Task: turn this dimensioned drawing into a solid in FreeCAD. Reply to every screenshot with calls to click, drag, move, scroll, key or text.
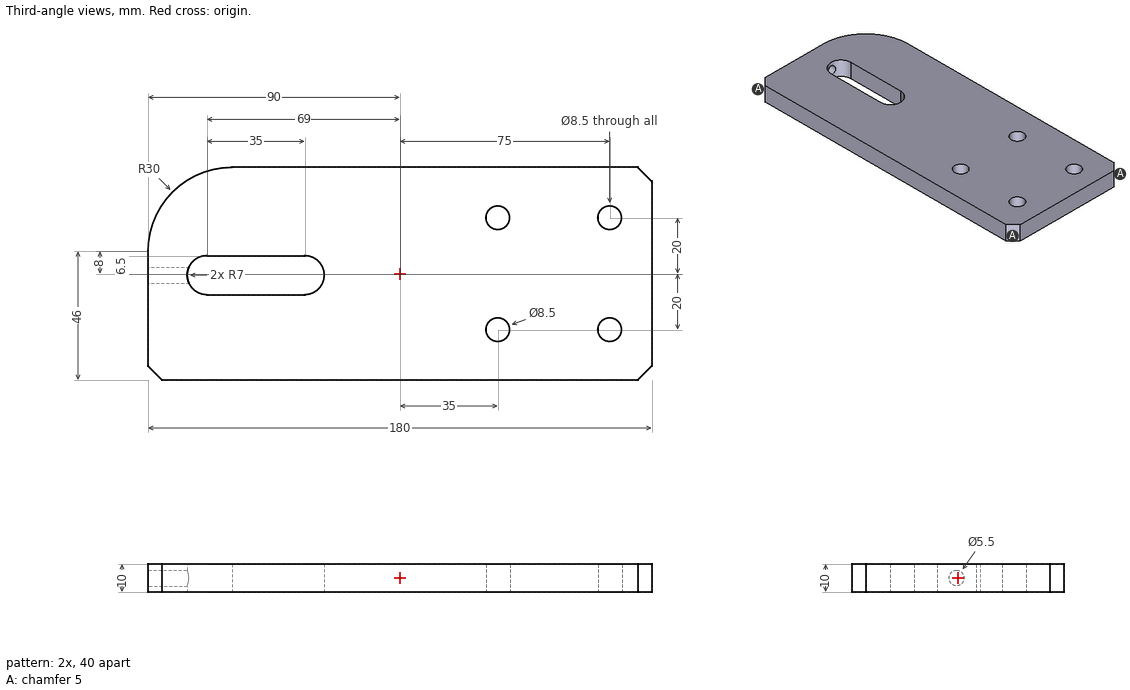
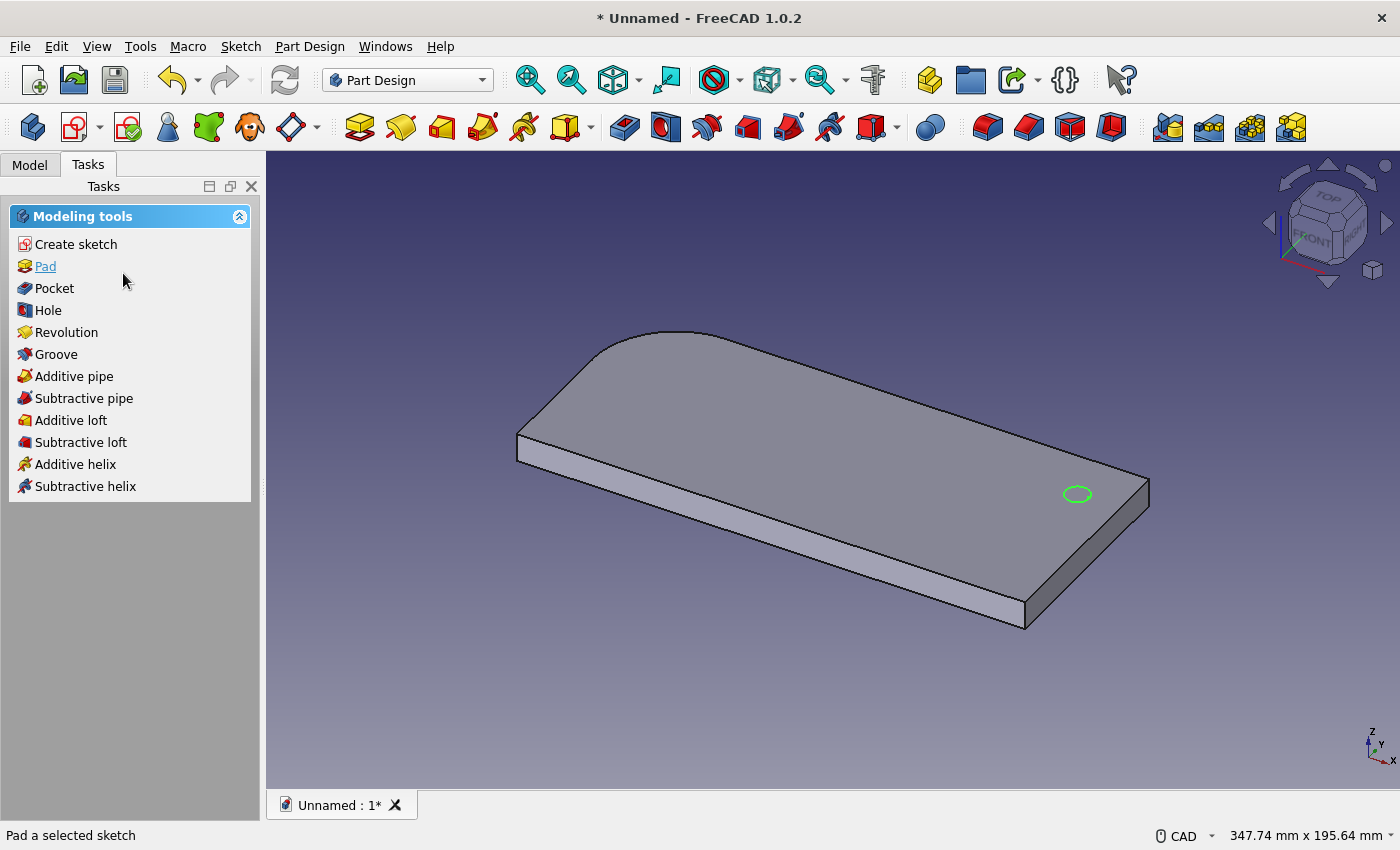
click(666, 128)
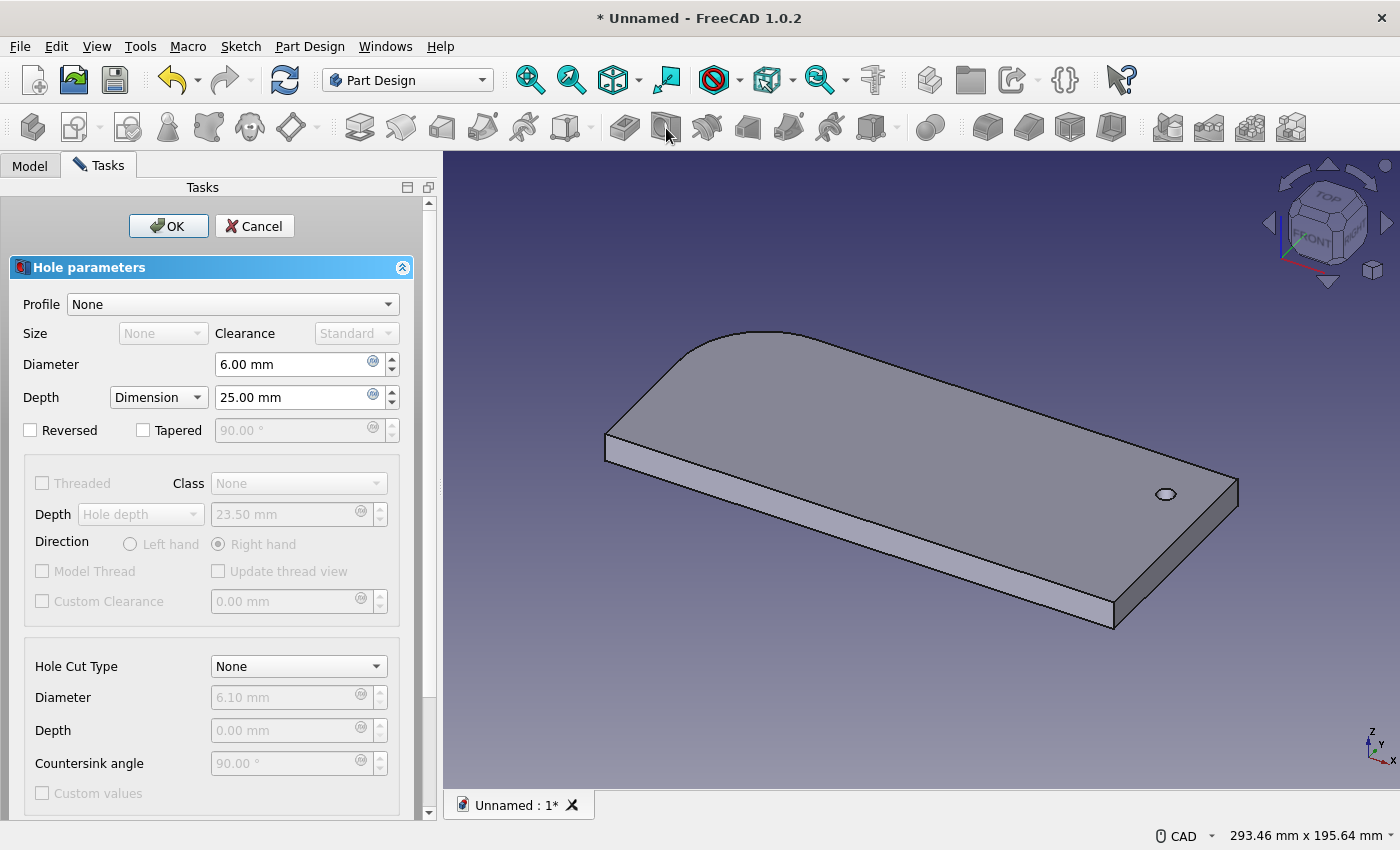
triple_click(300, 364)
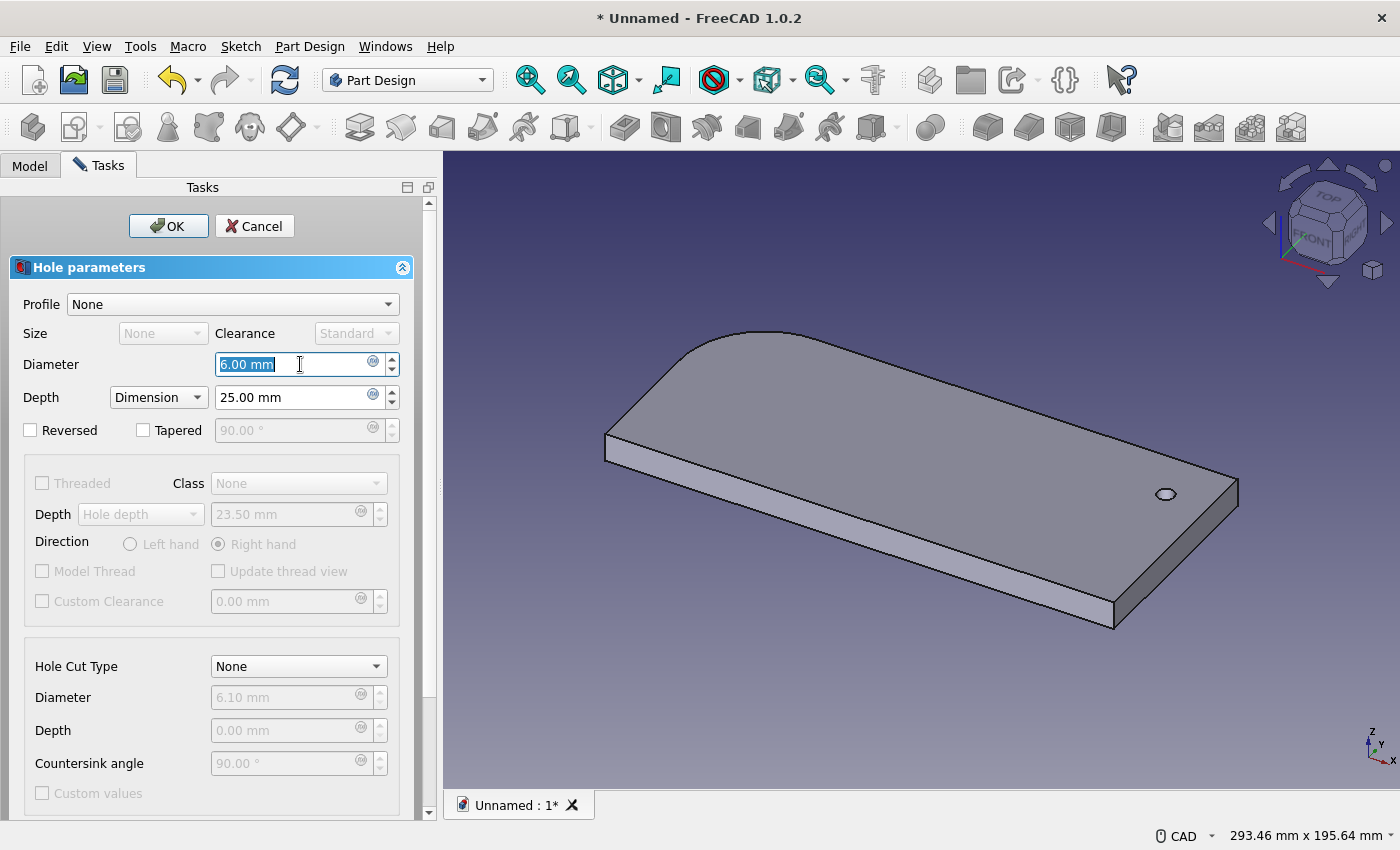
text(8.5)
key(Tab)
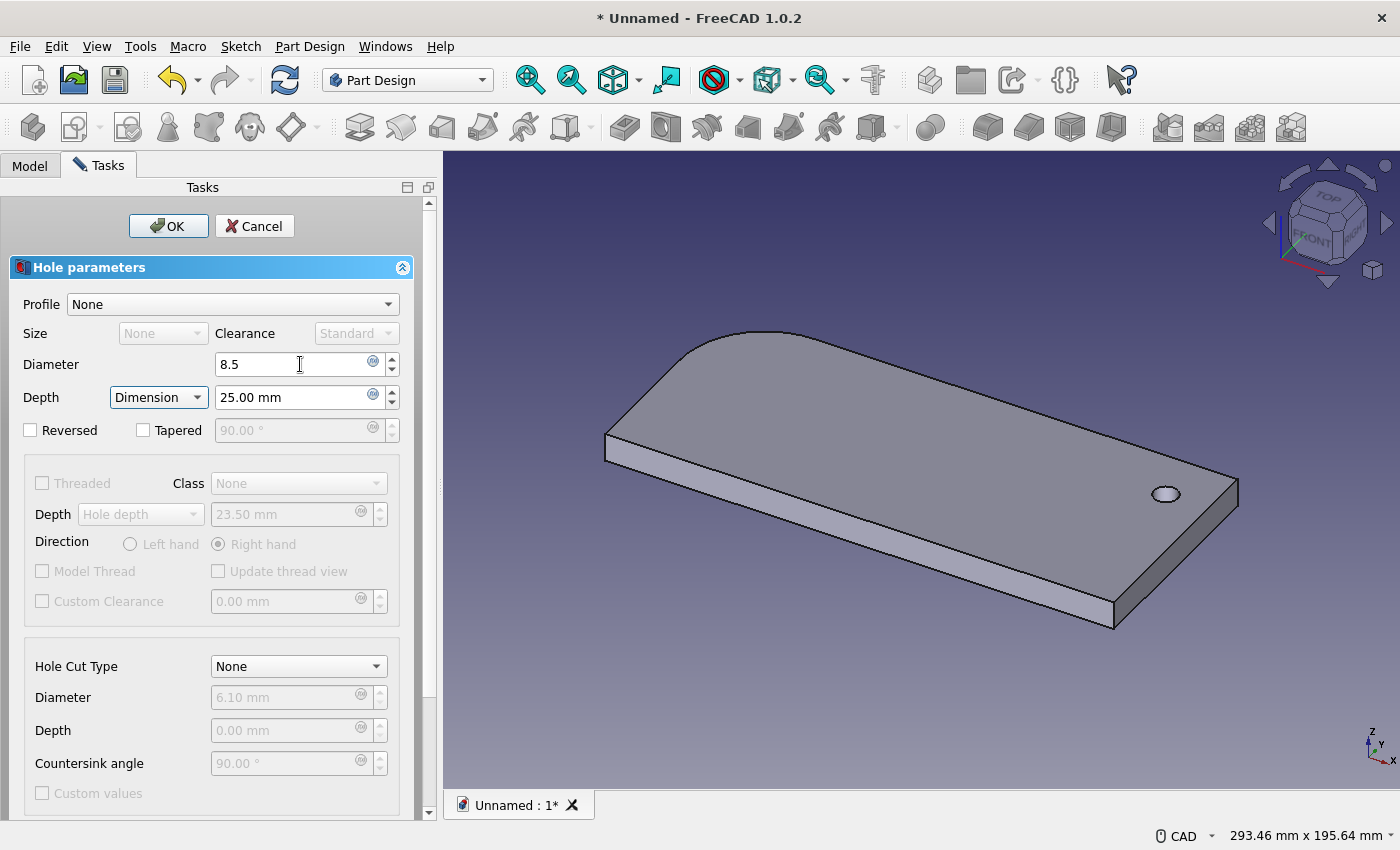
click(160, 398)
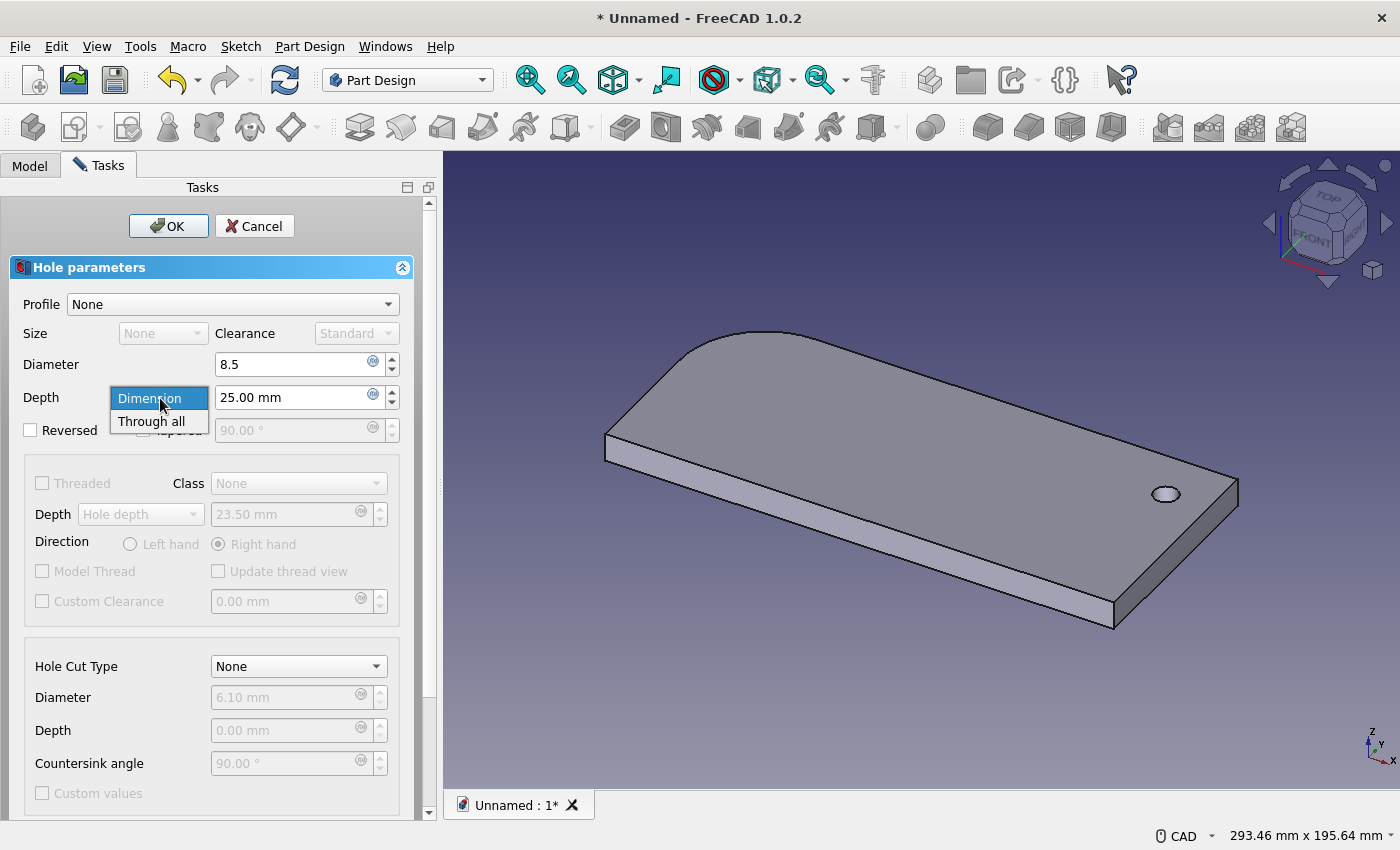
click(158, 422)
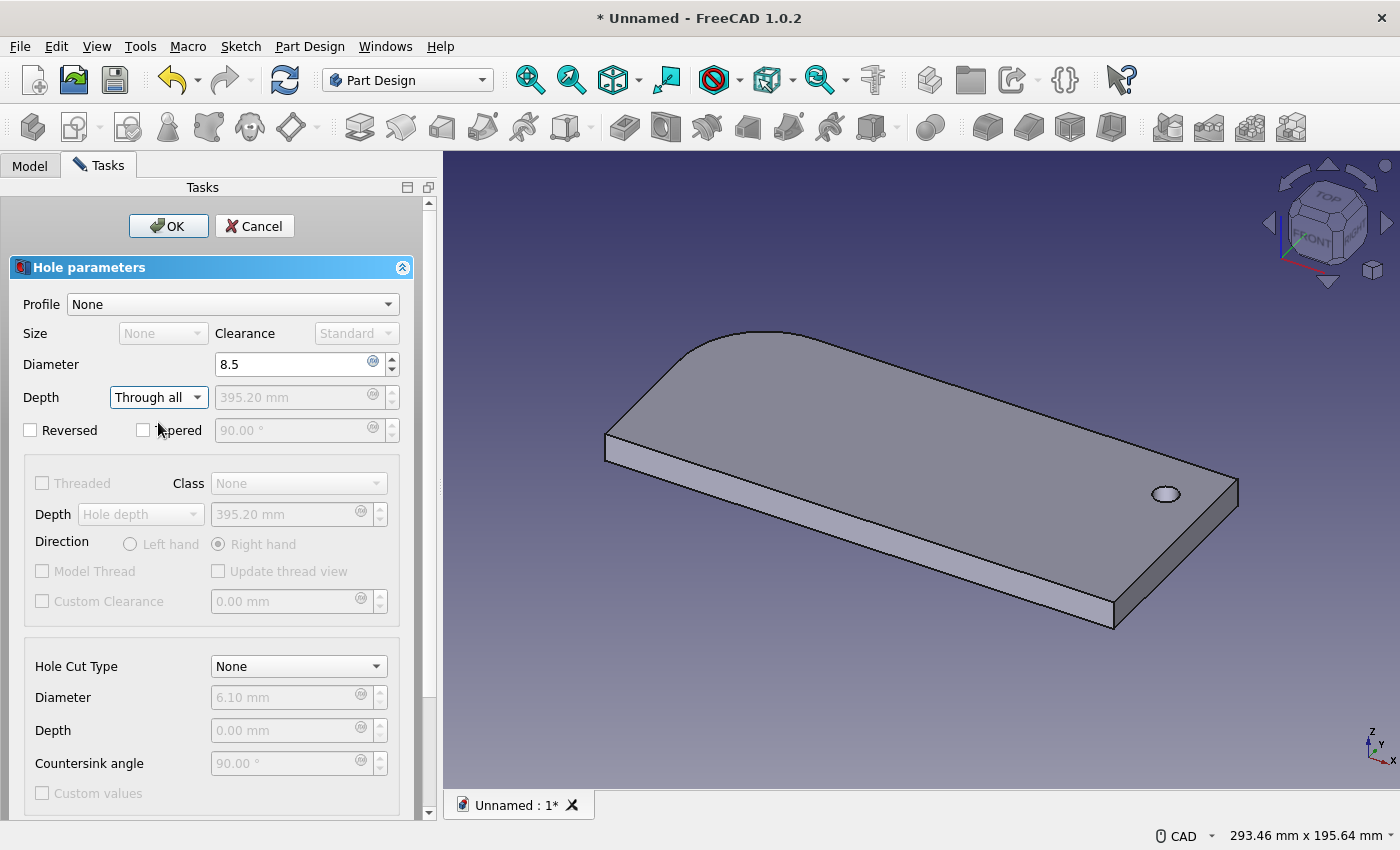
click(169, 226)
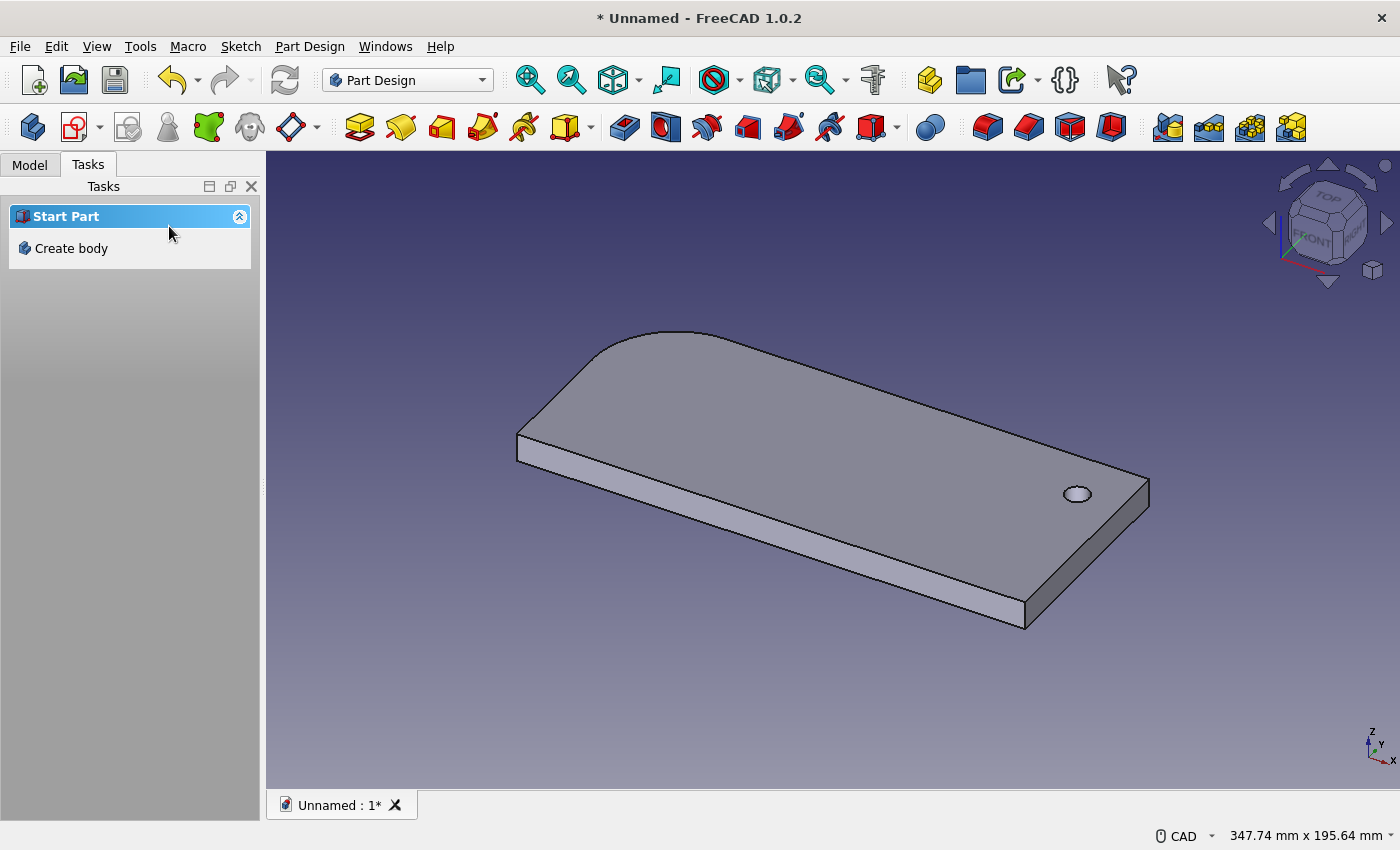
click(30, 164)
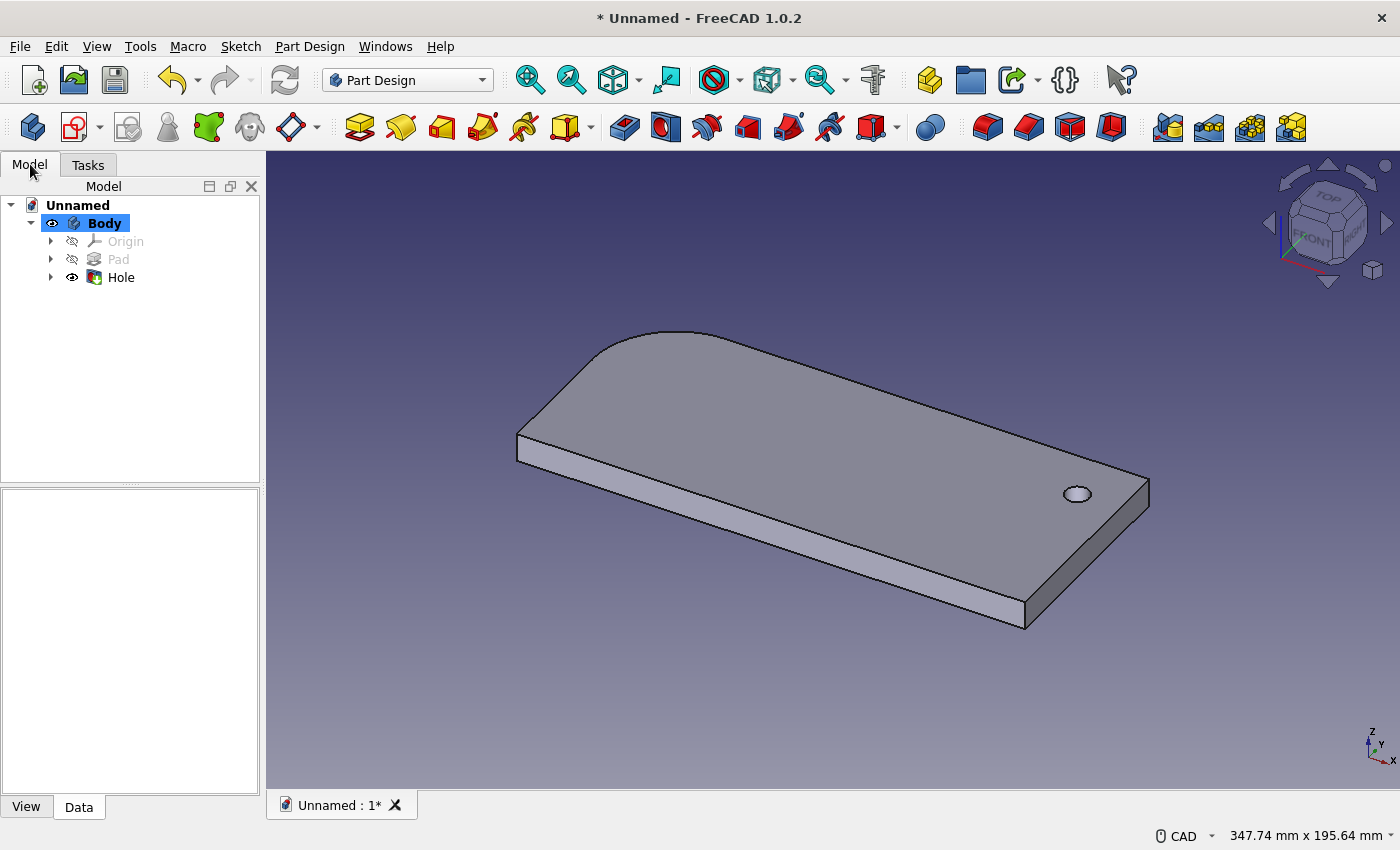
click(117, 277)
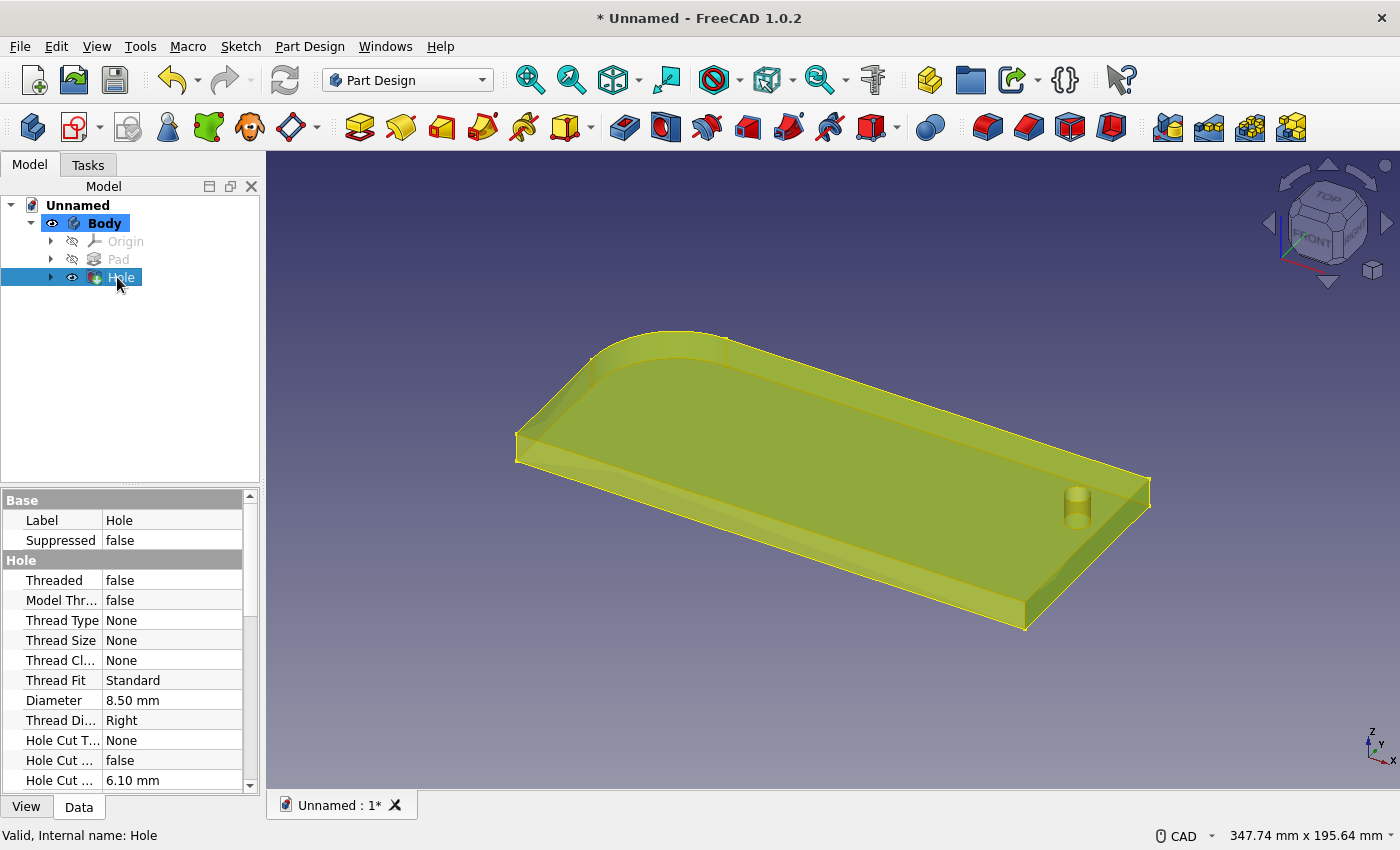
click(1209, 128)